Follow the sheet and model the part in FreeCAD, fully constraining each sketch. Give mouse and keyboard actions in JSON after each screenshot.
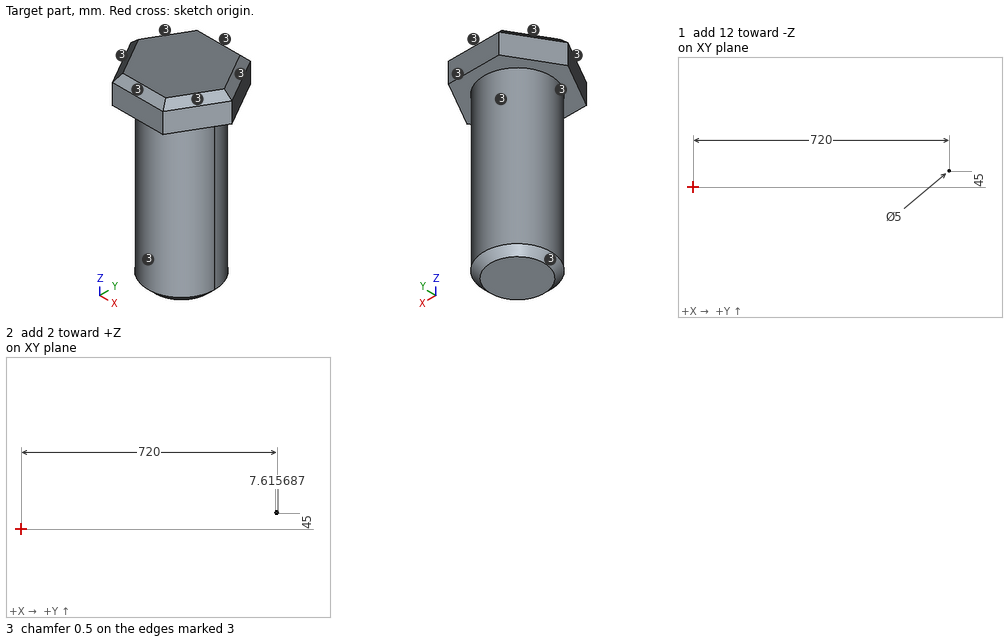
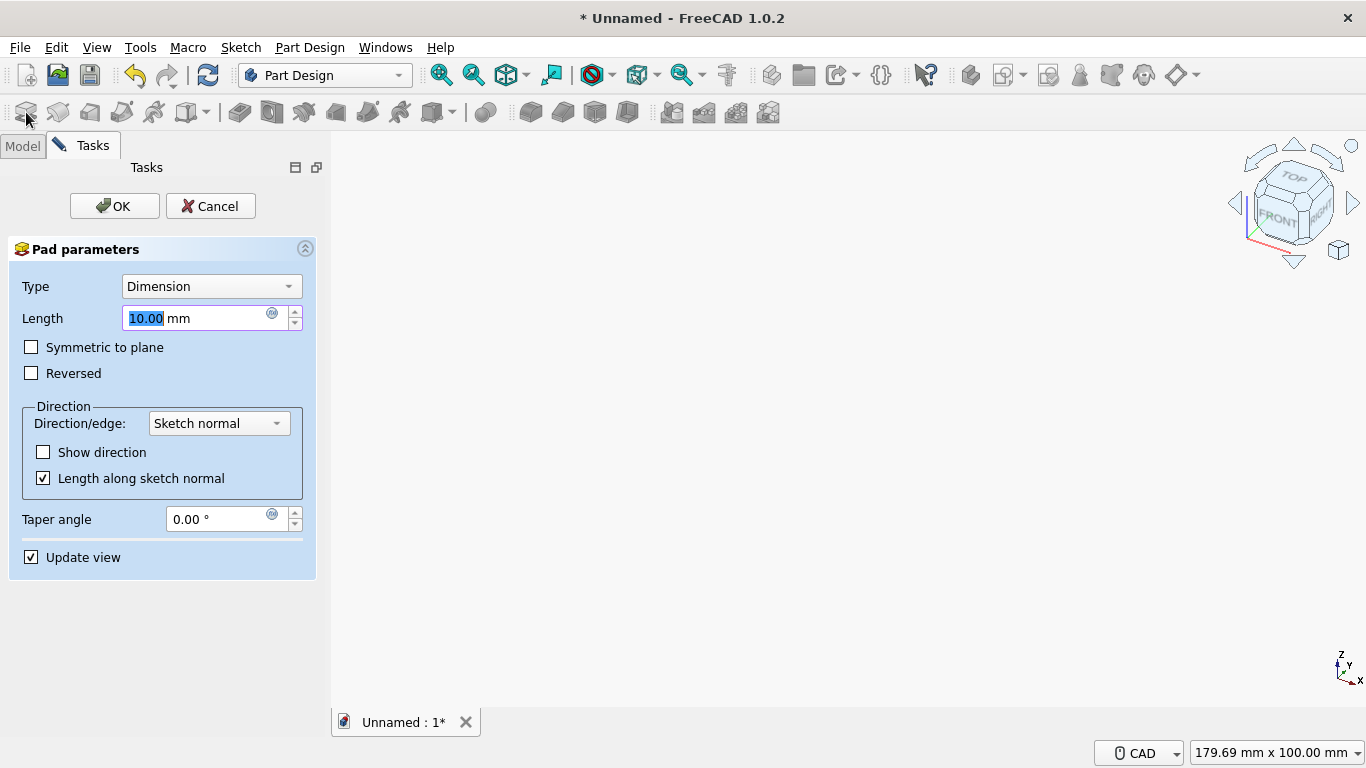
{"action": "type", "text": "12"}
{"action": "key", "text": "Tab"}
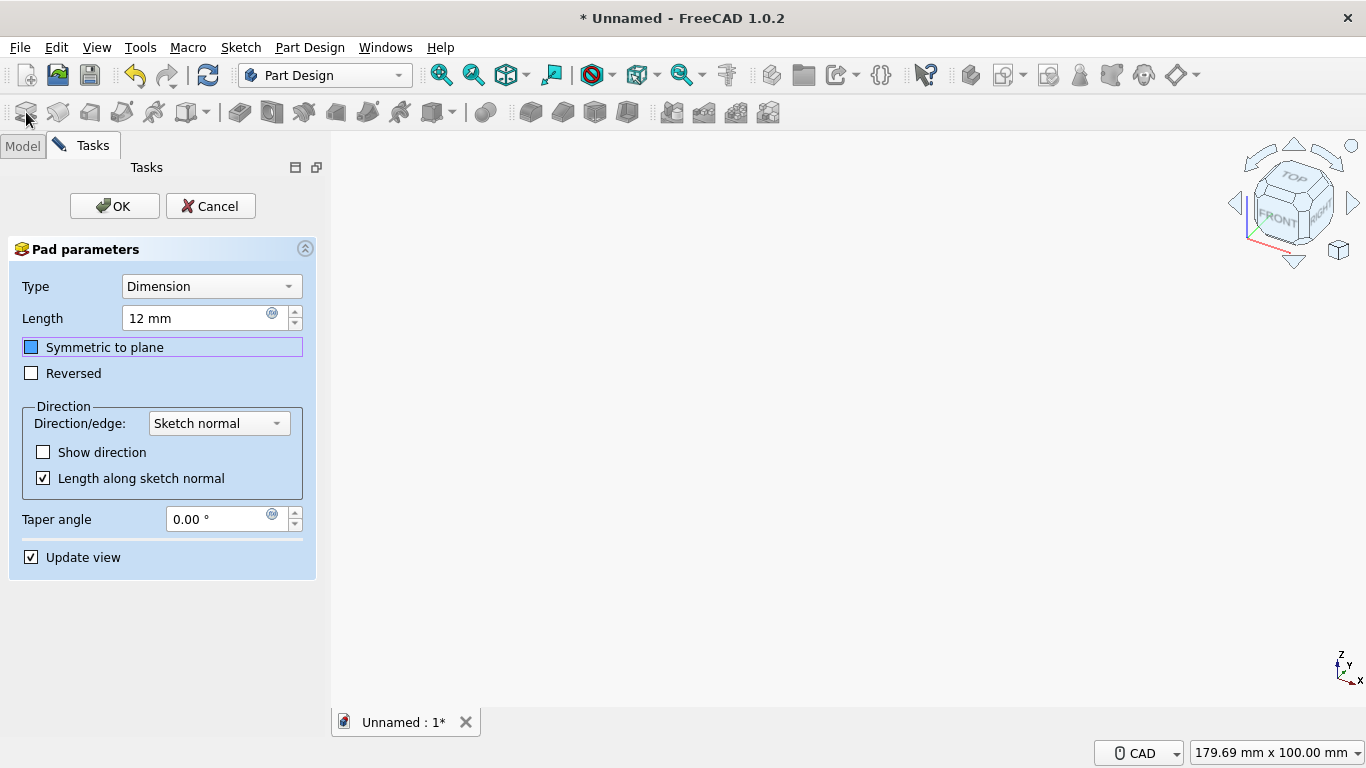
{"action": "left_click", "coordinate": [30, 373]}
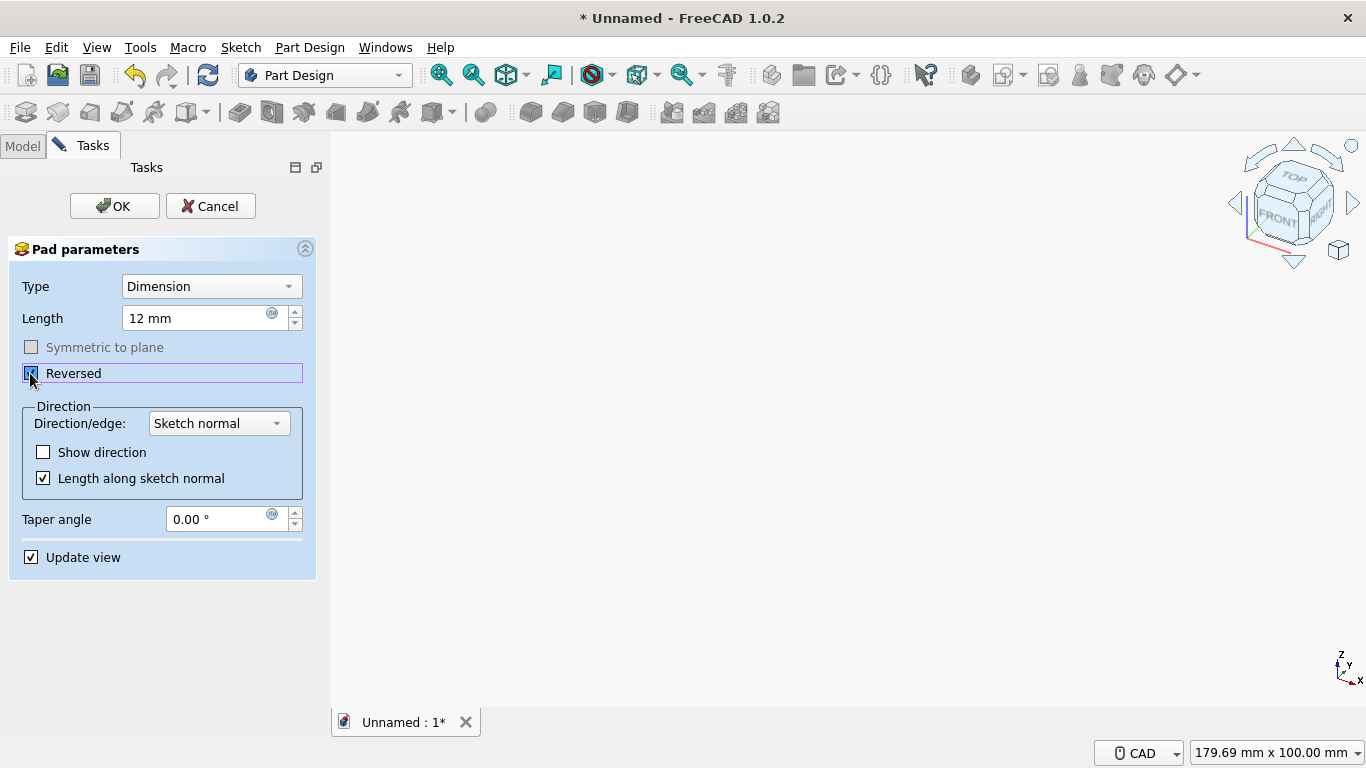
{"action": "left_click", "coordinate": [115, 206]}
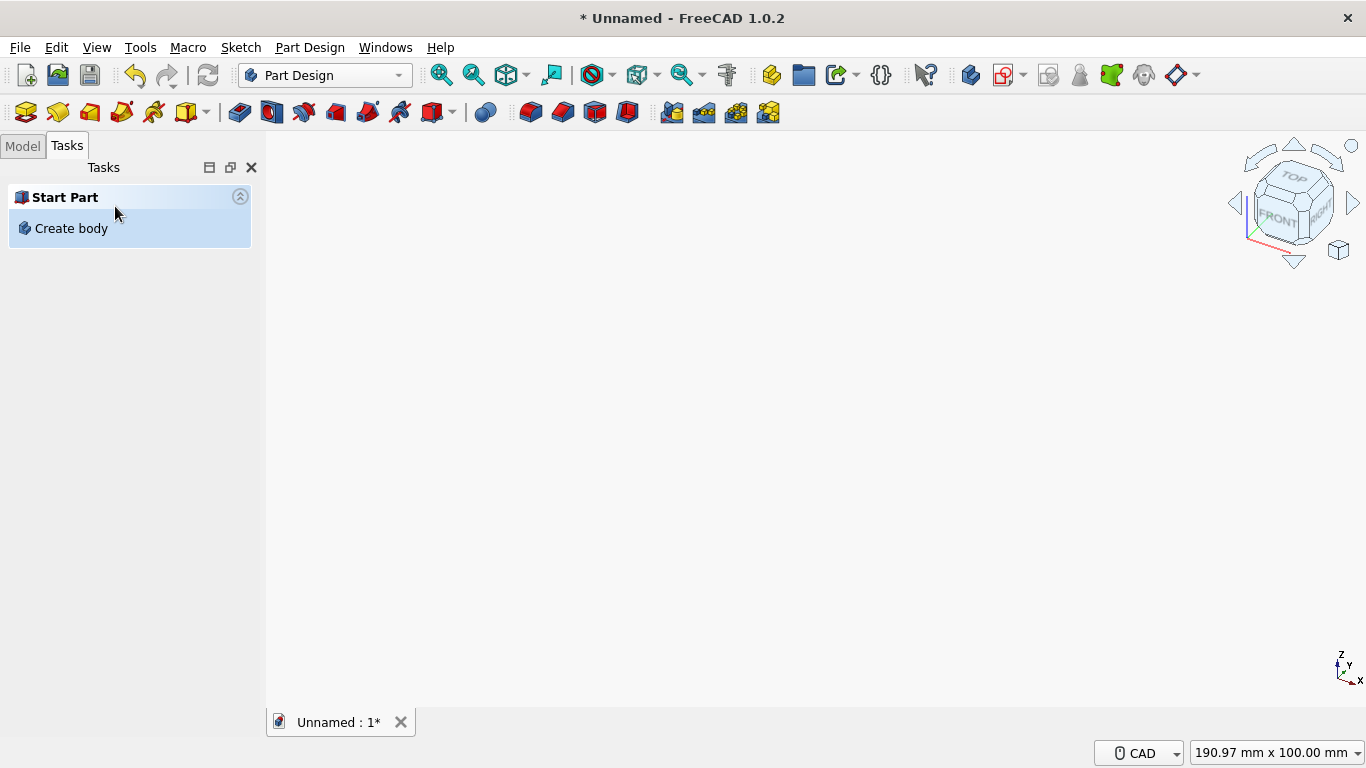
{"action": "left_click", "coordinate": [442, 76]}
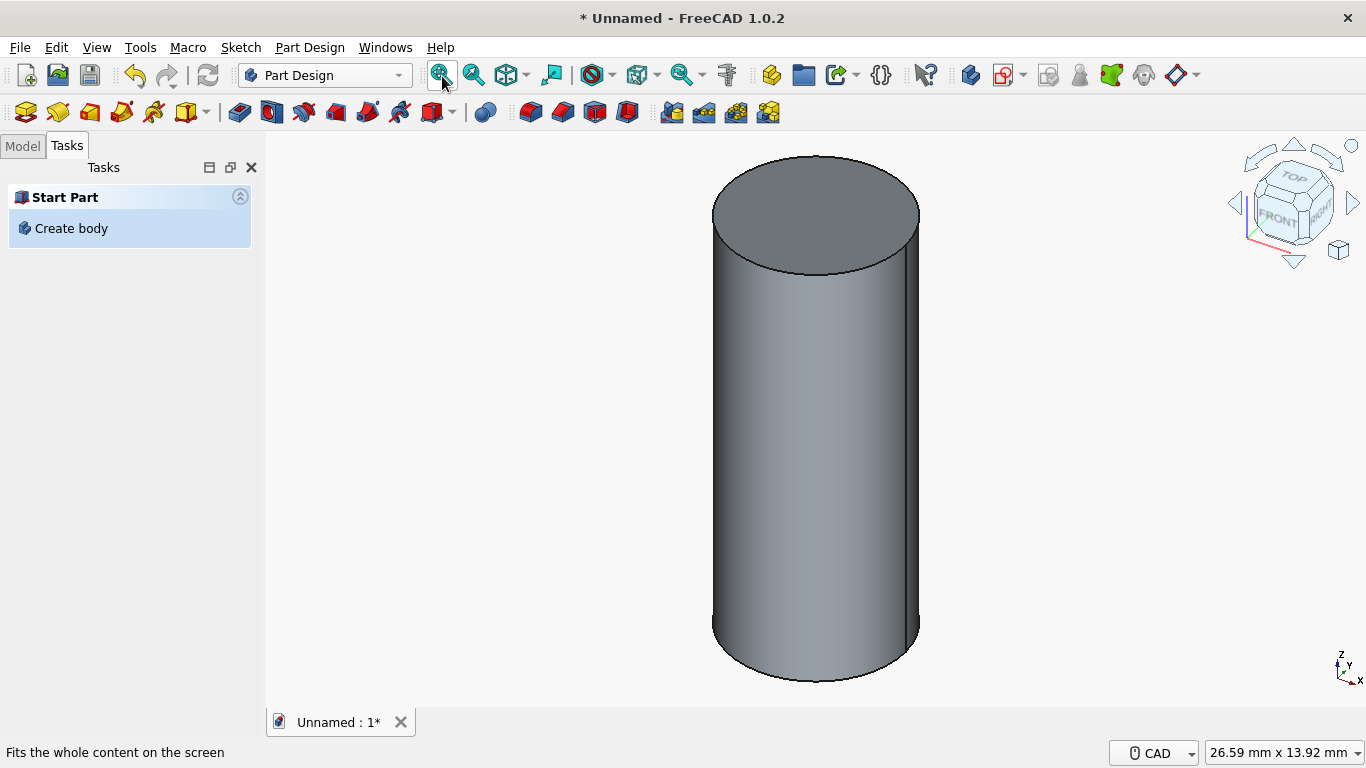
{"action": "left_click", "coordinate": [1004, 76]}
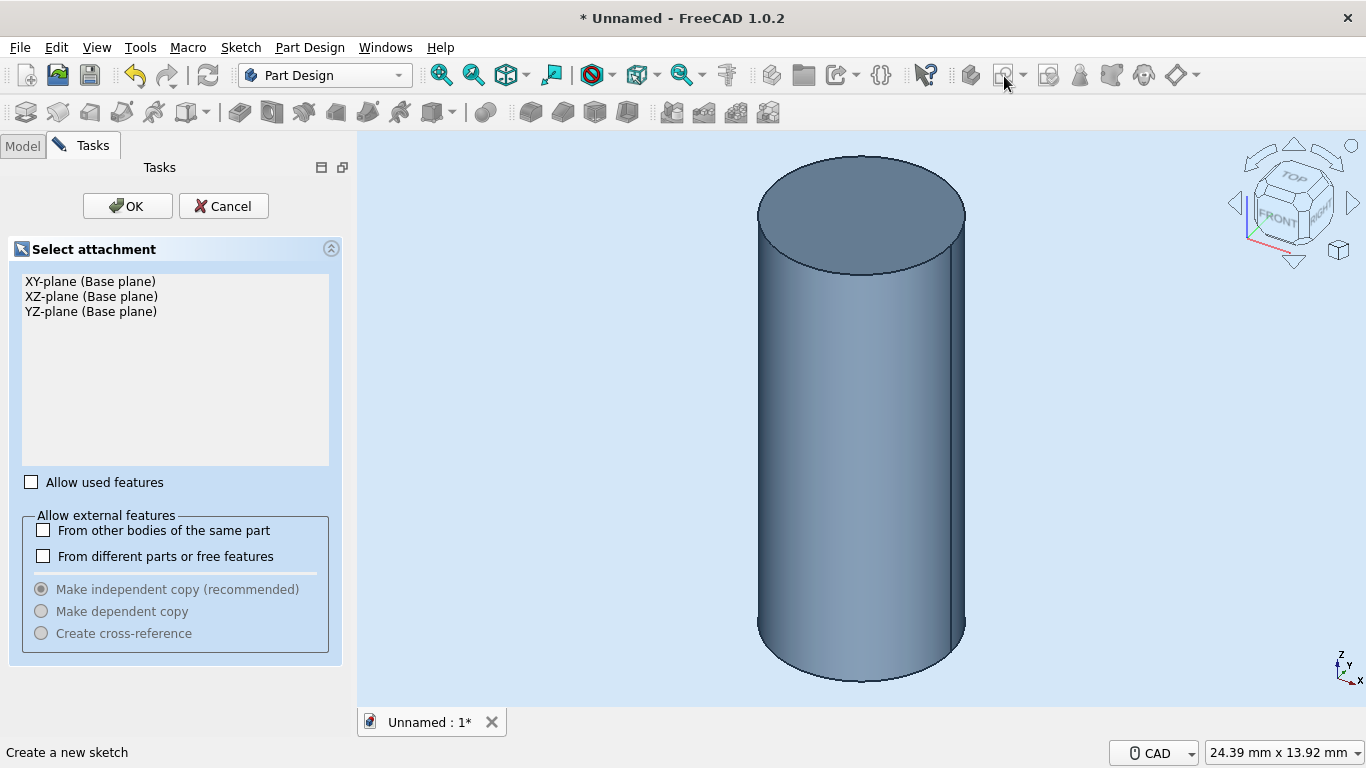
{"action": "left_click", "coordinate": [82, 282]}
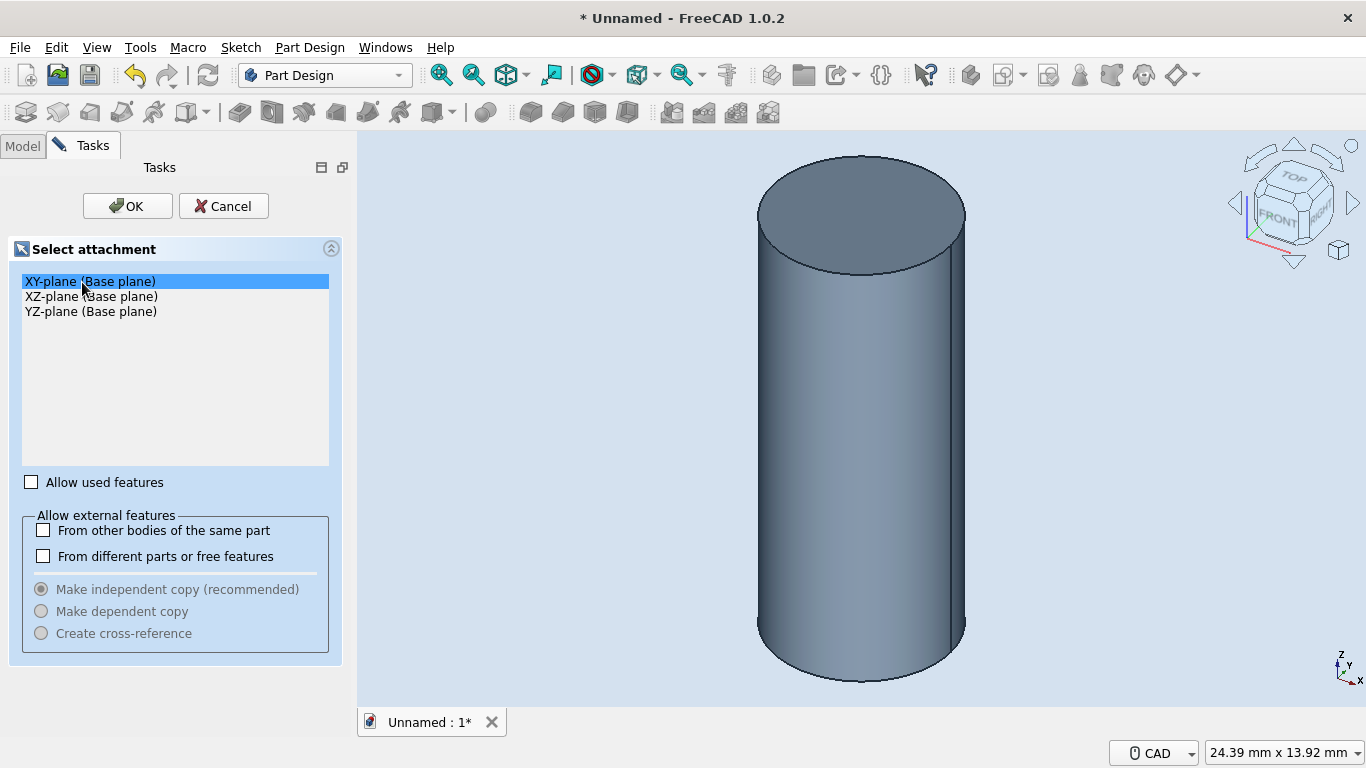
{"action": "left_click", "coordinate": [128, 206]}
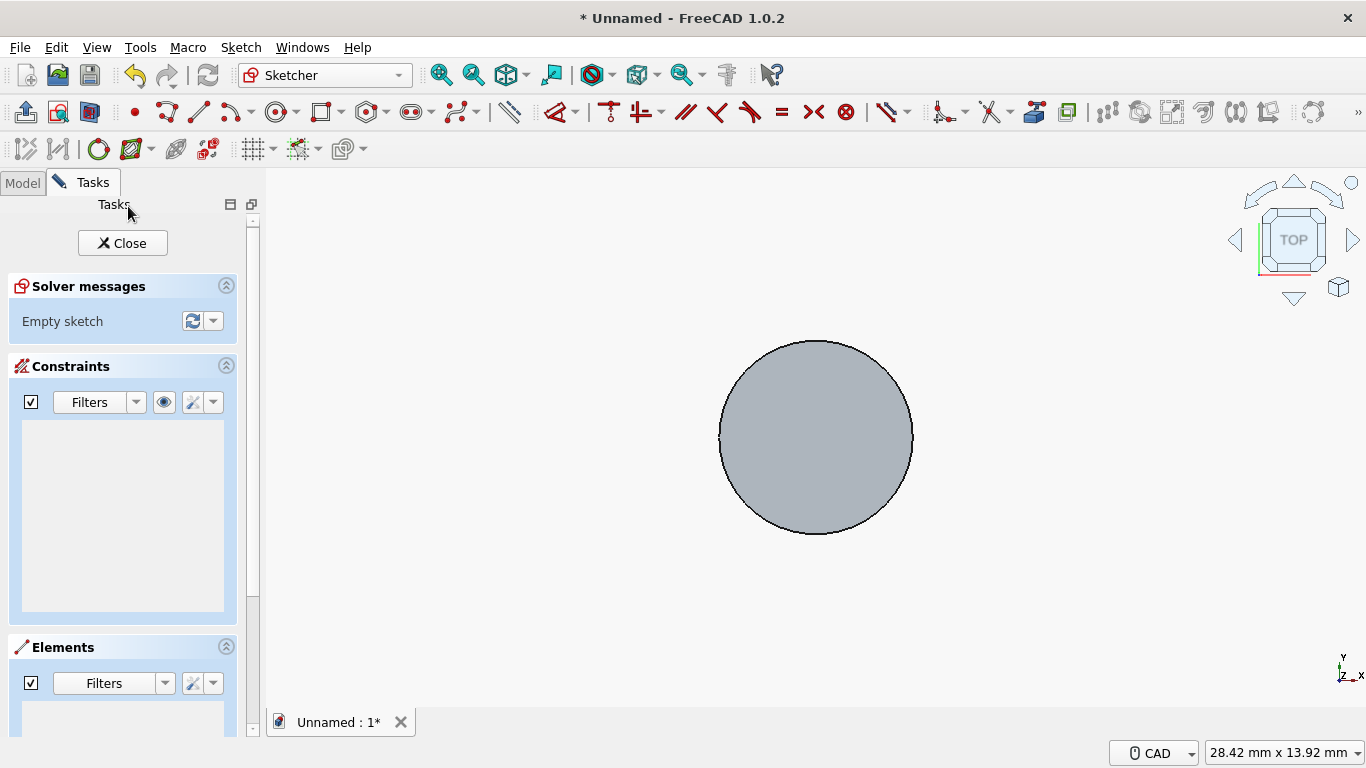
{"action": "left_click", "coordinate": [366, 112]}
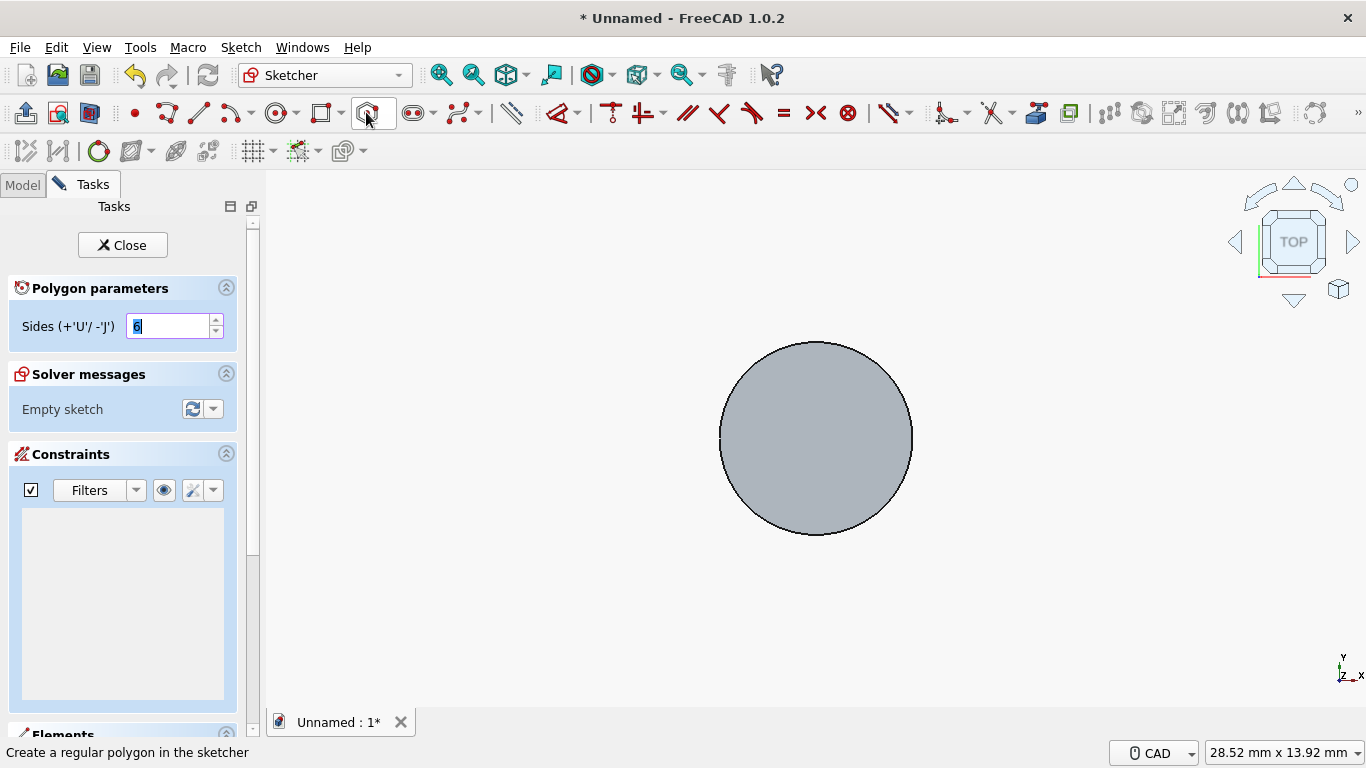
{"action": "left_click", "coordinate": [816, 439]}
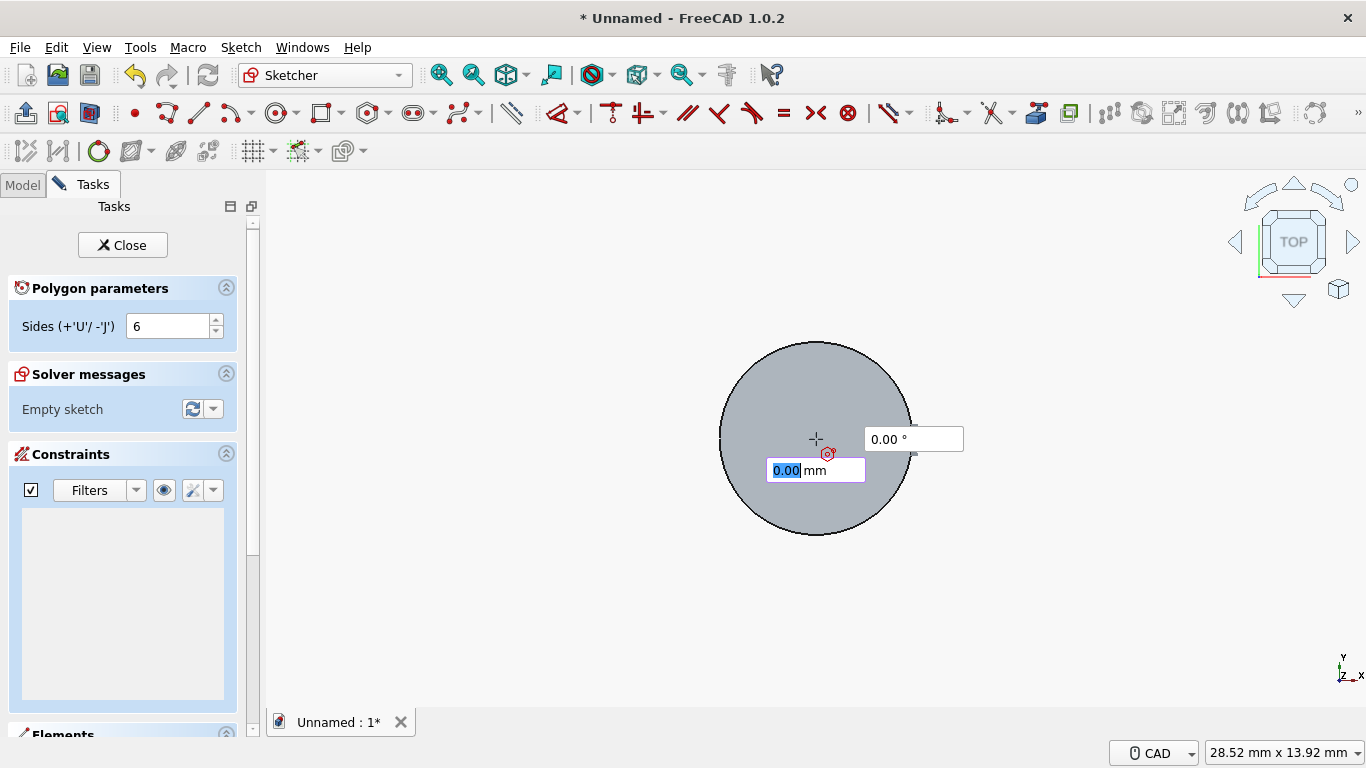
{"action": "left_click", "coordinate": [963, 439]}
{"action": "right_click", "coordinate": [963, 439]}